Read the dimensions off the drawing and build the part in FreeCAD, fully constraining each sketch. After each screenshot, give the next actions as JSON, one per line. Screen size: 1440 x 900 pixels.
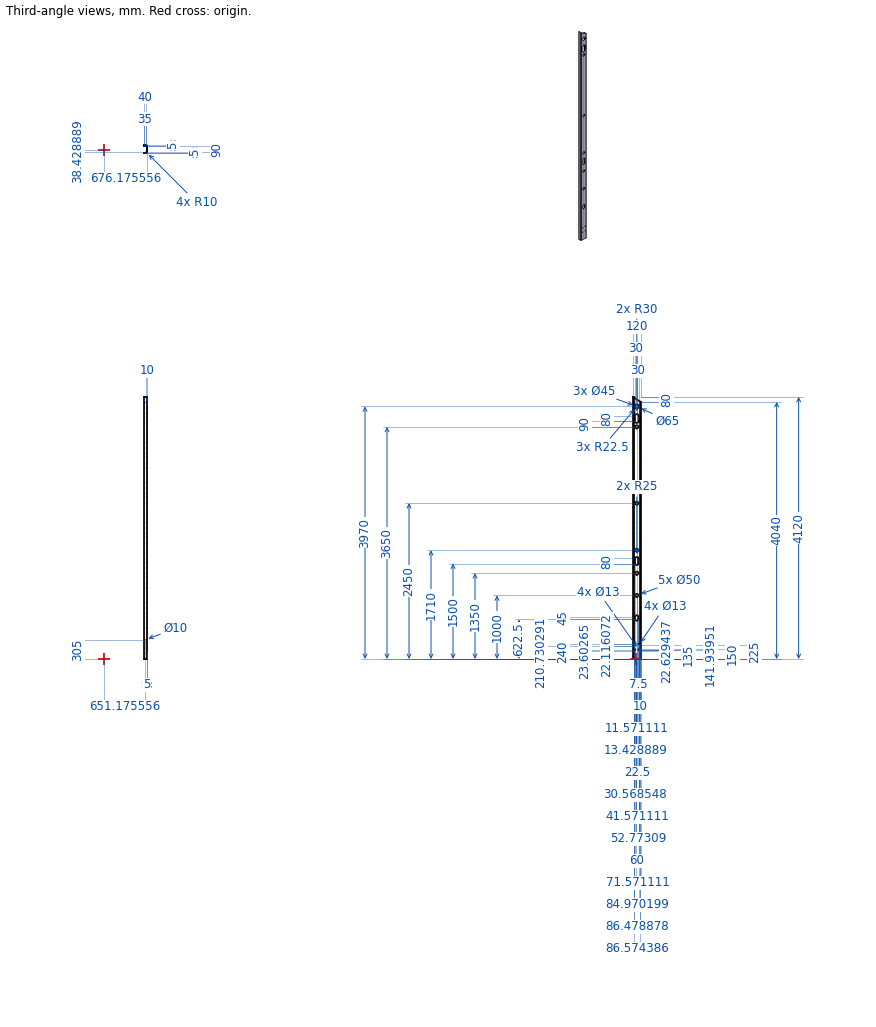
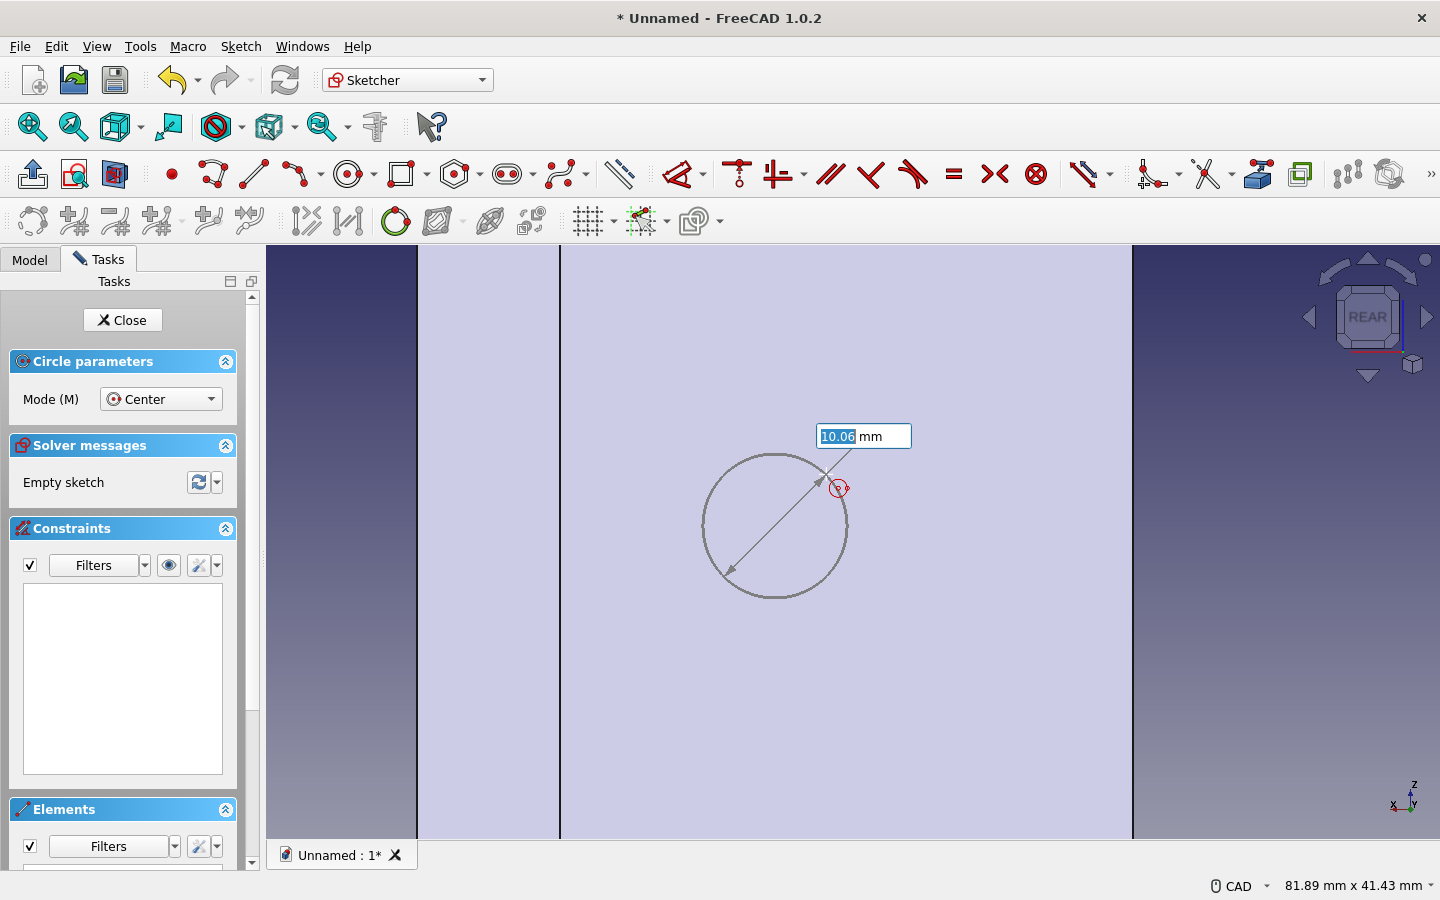
{"action": "type", "text": "10"}
{"action": "key", "text": "Return"}
{"action": "key", "text": "Escape"}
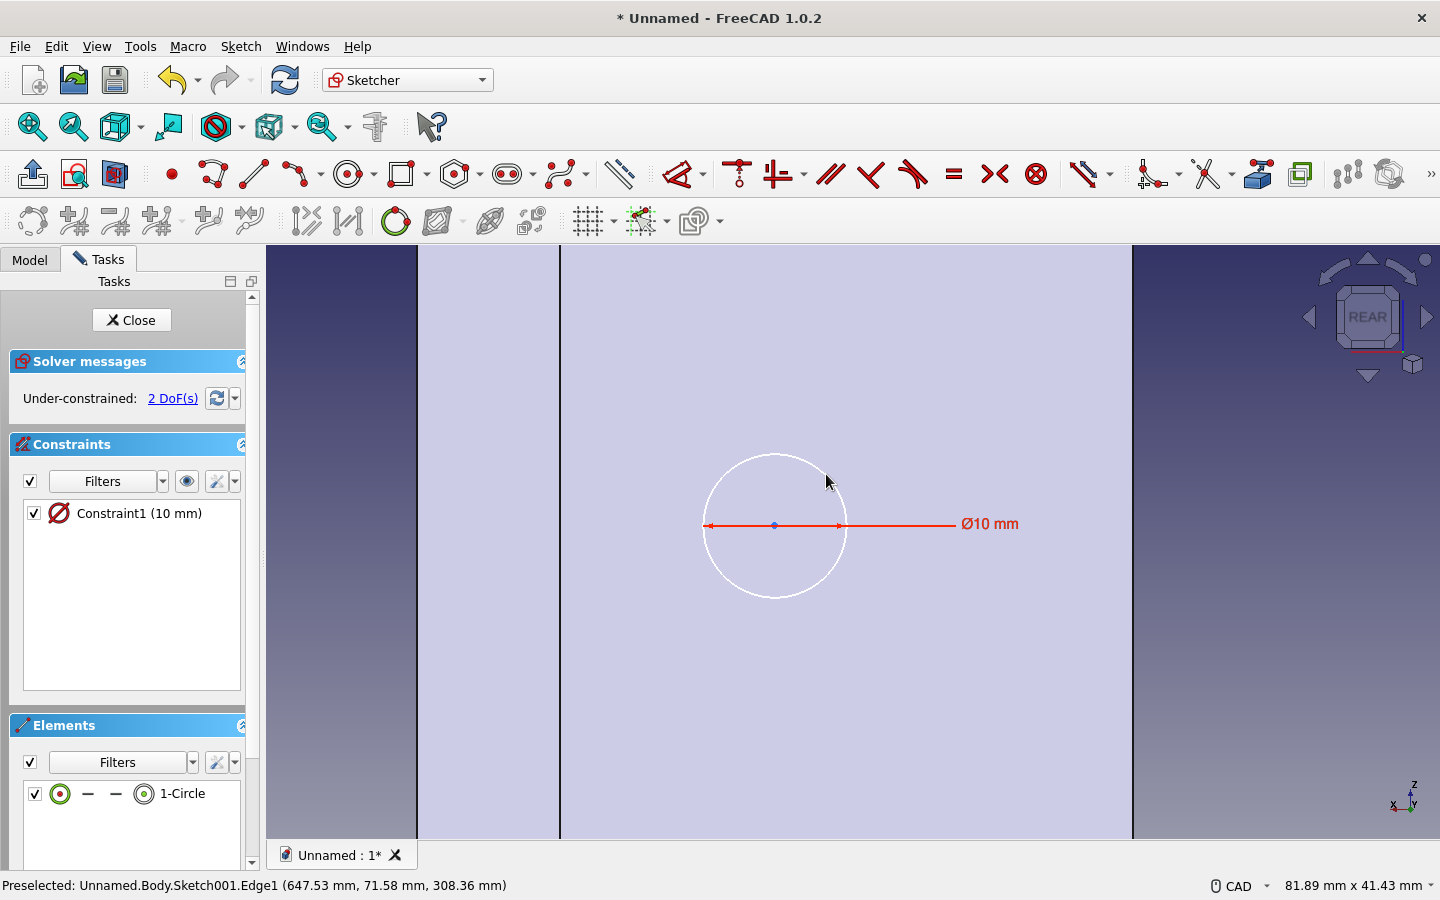
{"action": "left_click", "coordinate": [676, 174]}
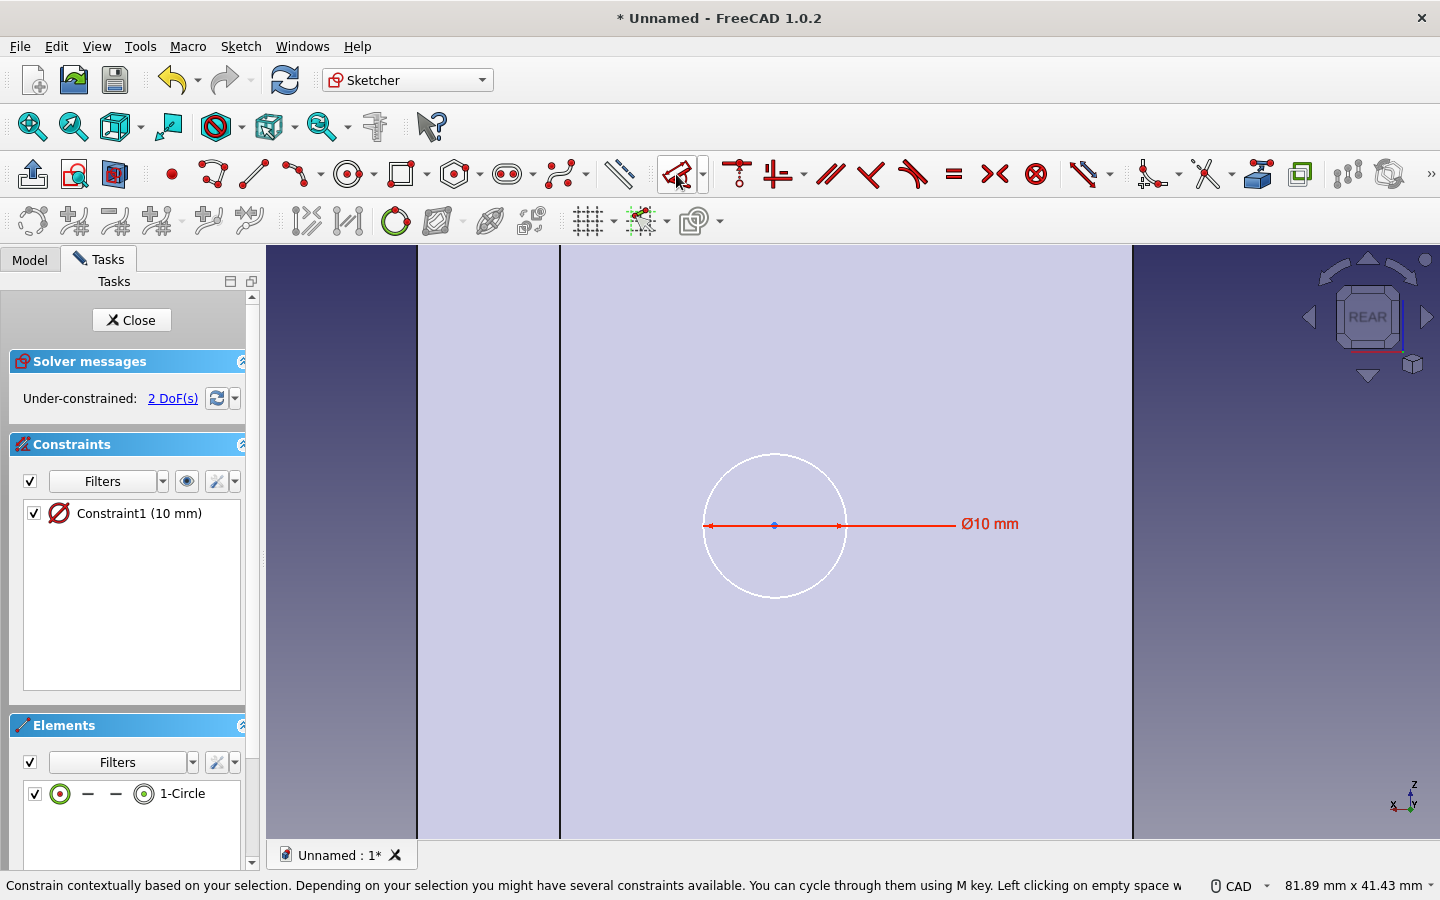
{"action": "left_click", "coordinate": [775, 526]}
{"action": "left_click", "coordinate": [741, 668]}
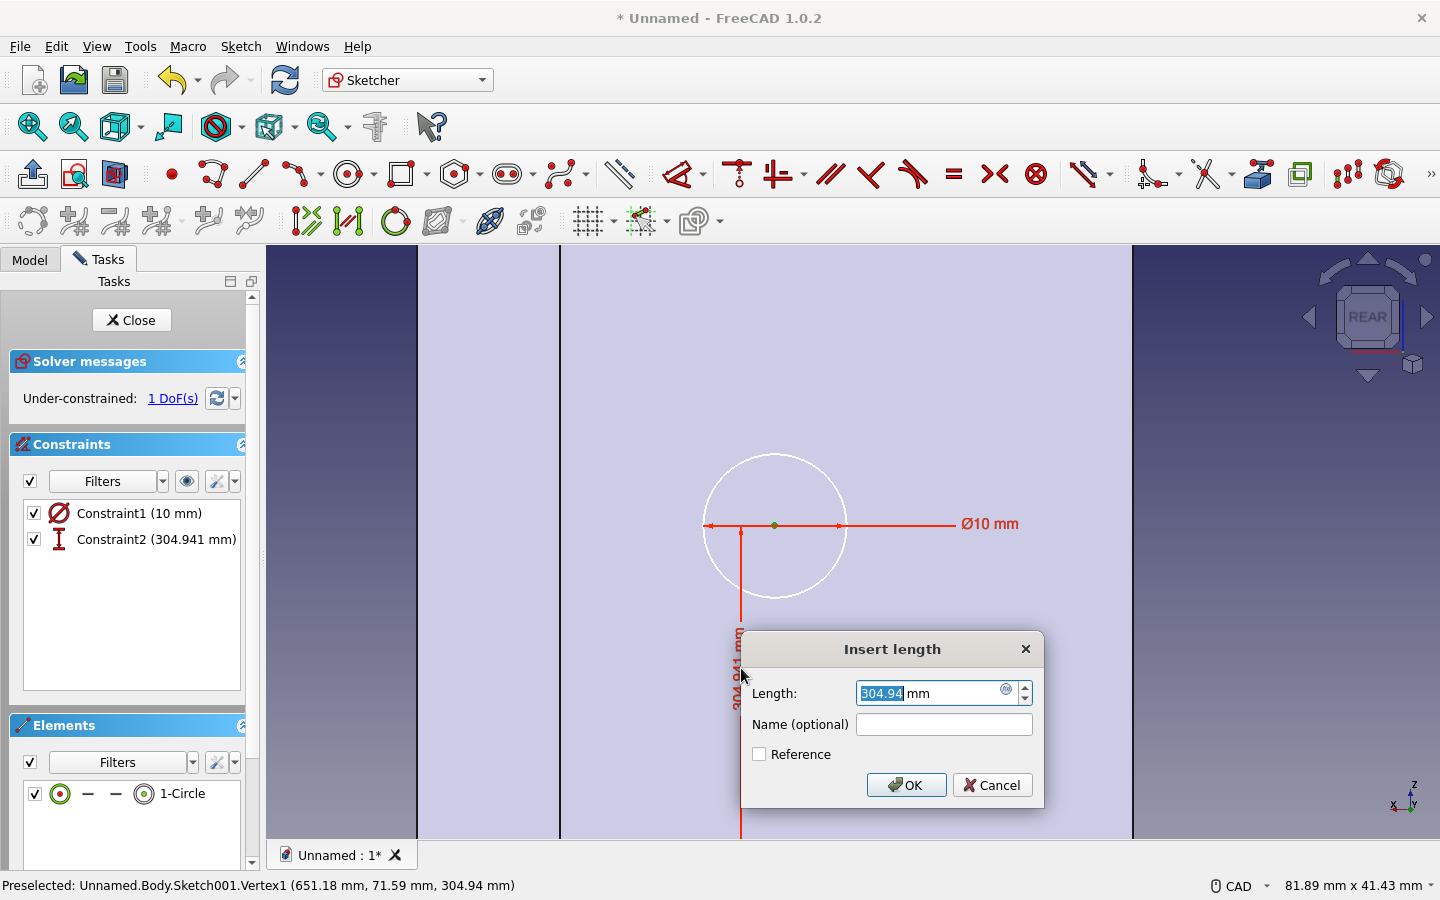
{"action": "type", "text": "305"}
{"action": "key", "text": "Return"}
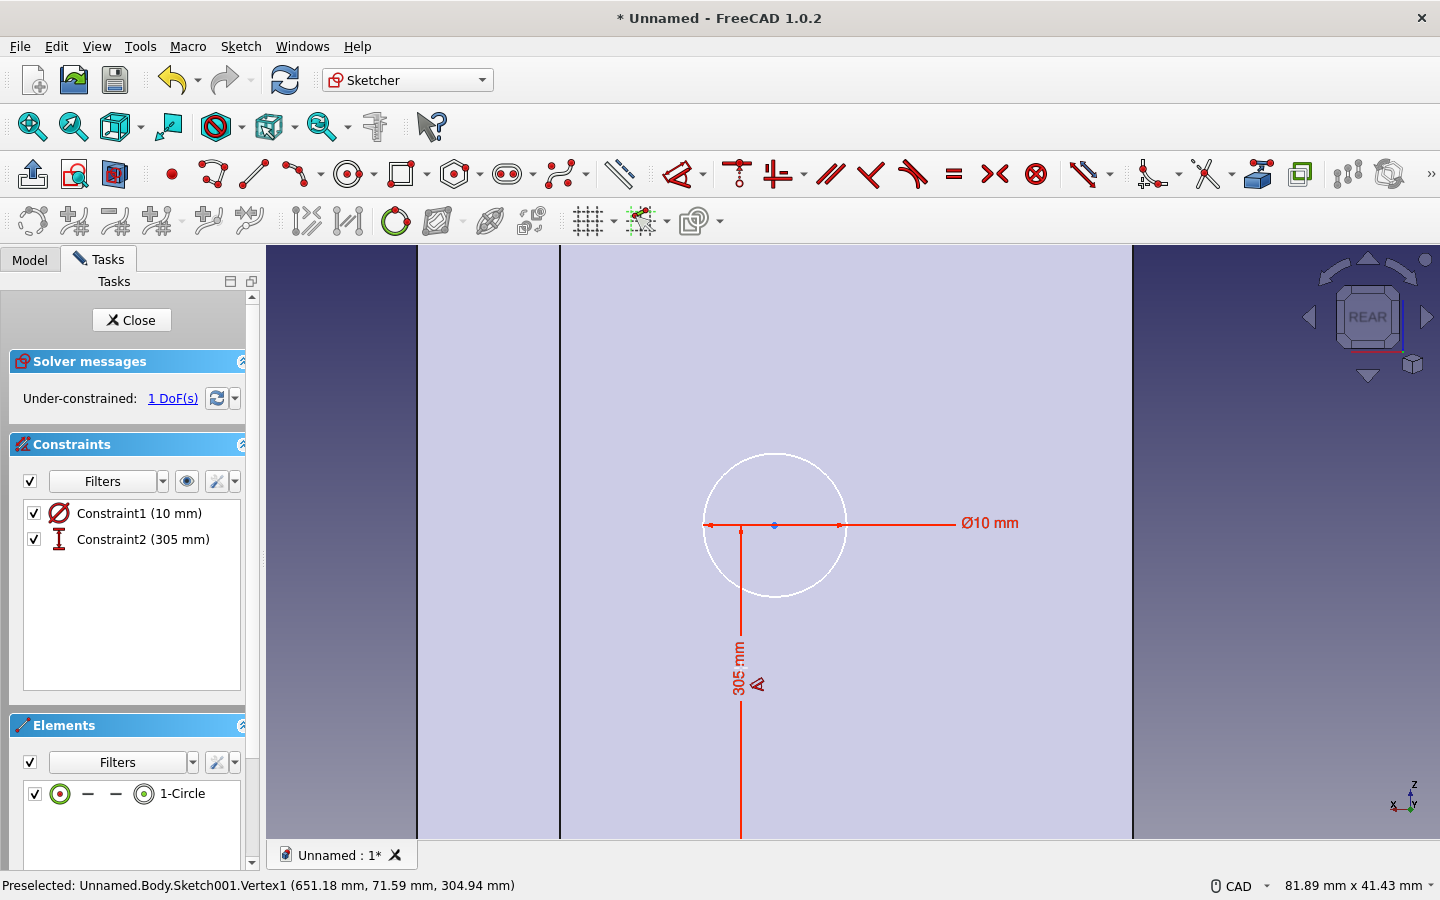
{"action": "left_click", "coordinate": [775, 525]}
{"action": "left_click", "coordinate": [1025, 491]}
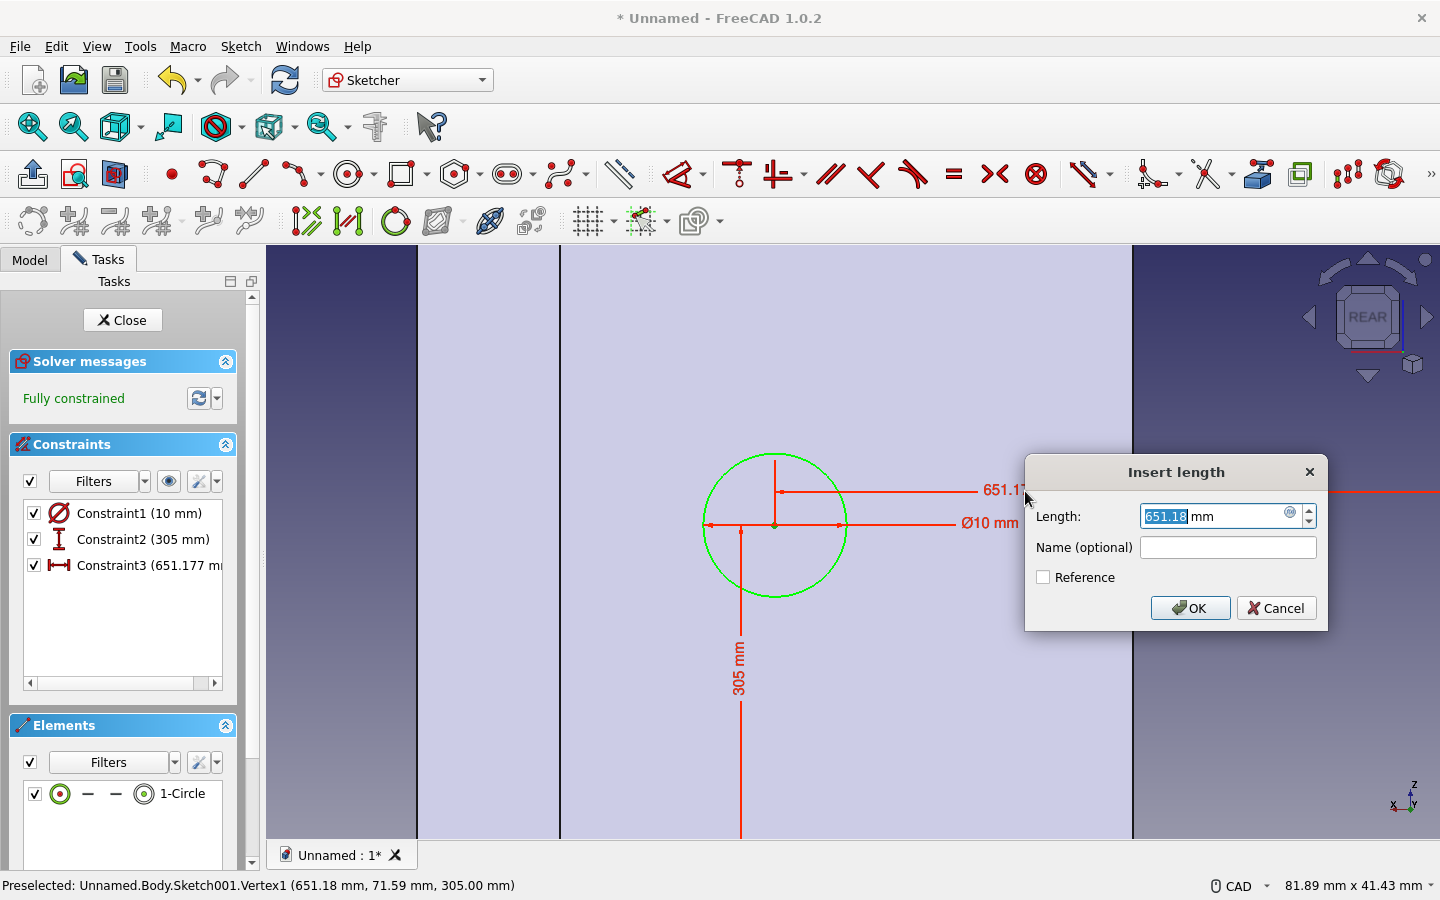
{"action": "type", "text": "651.175556"}
{"action": "key", "text": "Return"}
{"action": "key", "text": "Escape"}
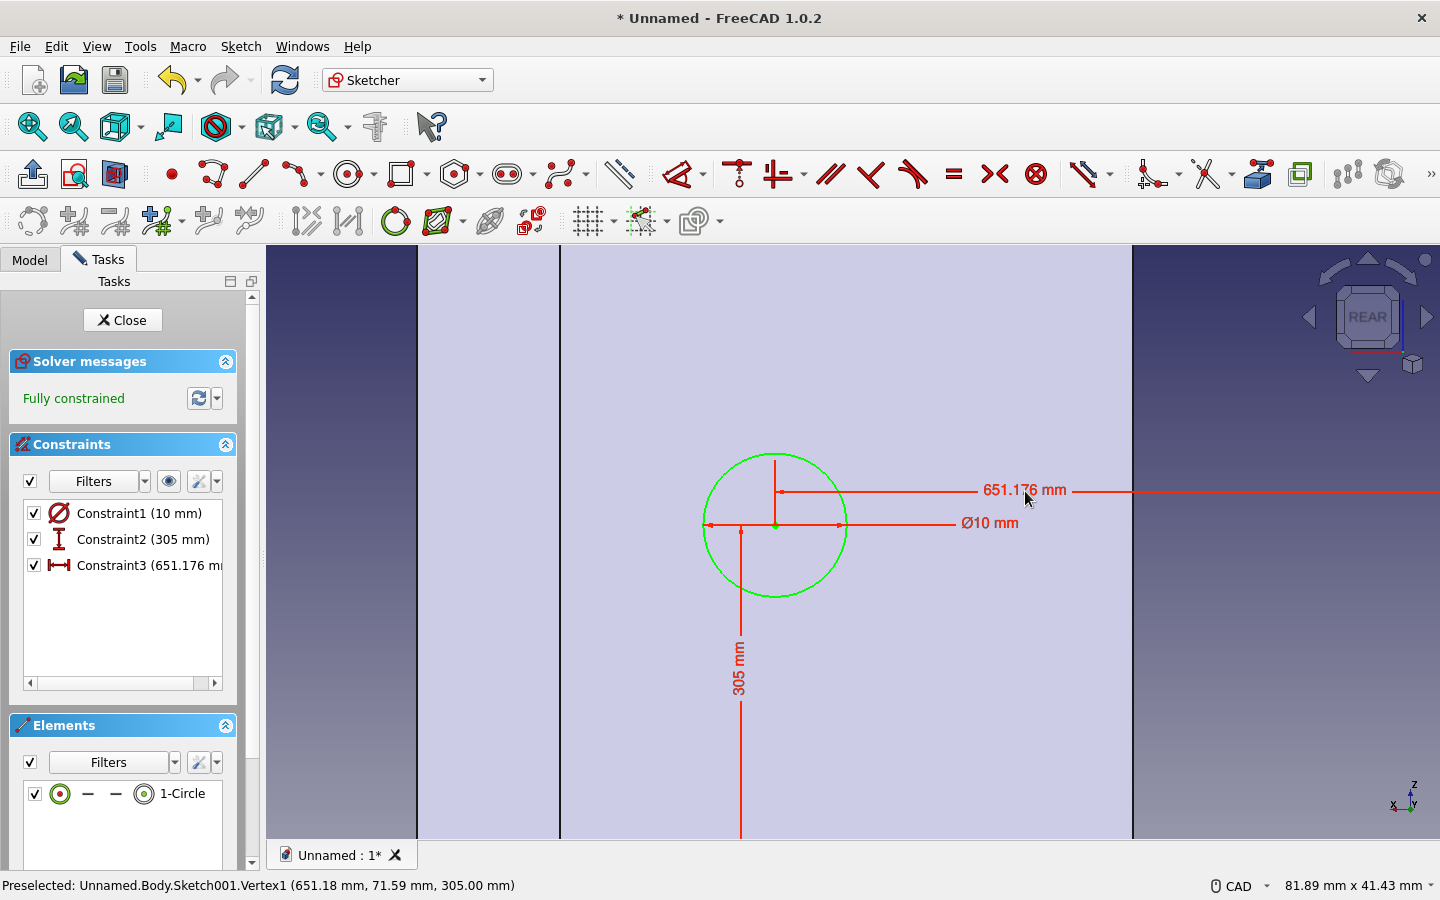
{"action": "left_click", "coordinate": [123, 320]}